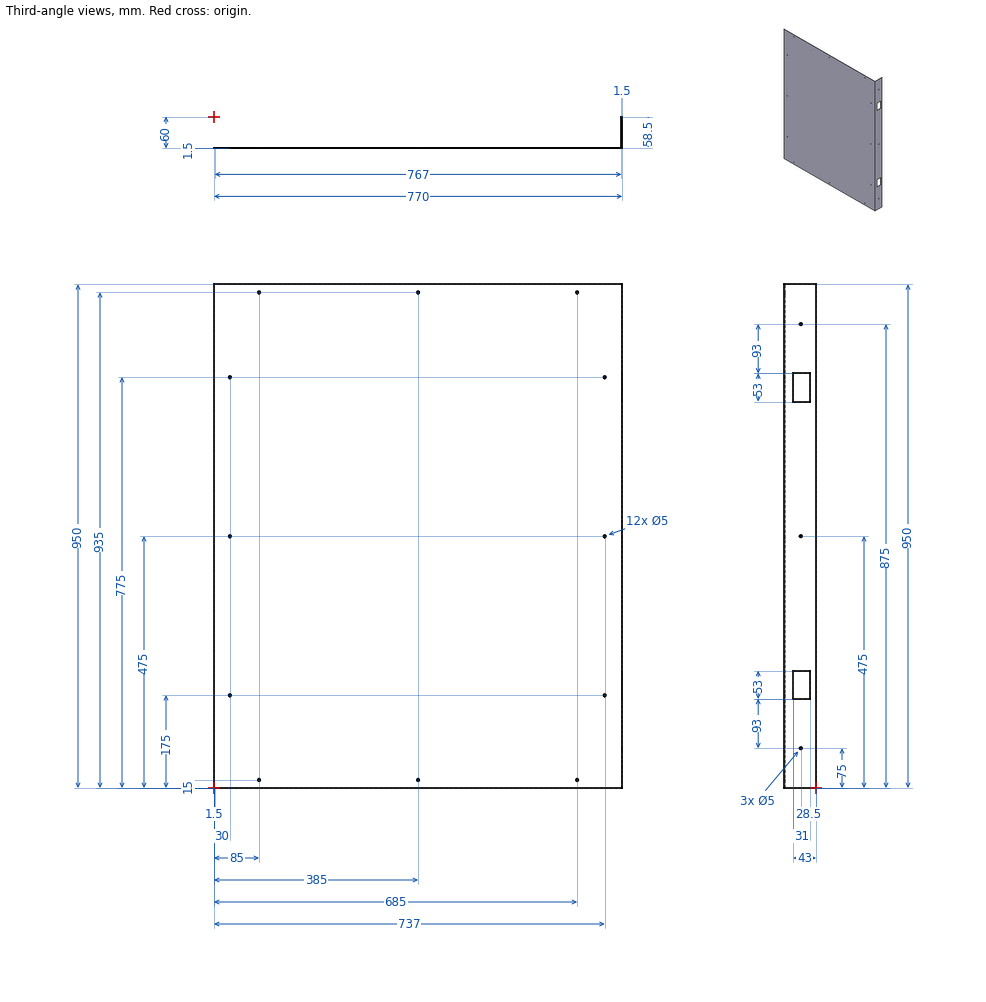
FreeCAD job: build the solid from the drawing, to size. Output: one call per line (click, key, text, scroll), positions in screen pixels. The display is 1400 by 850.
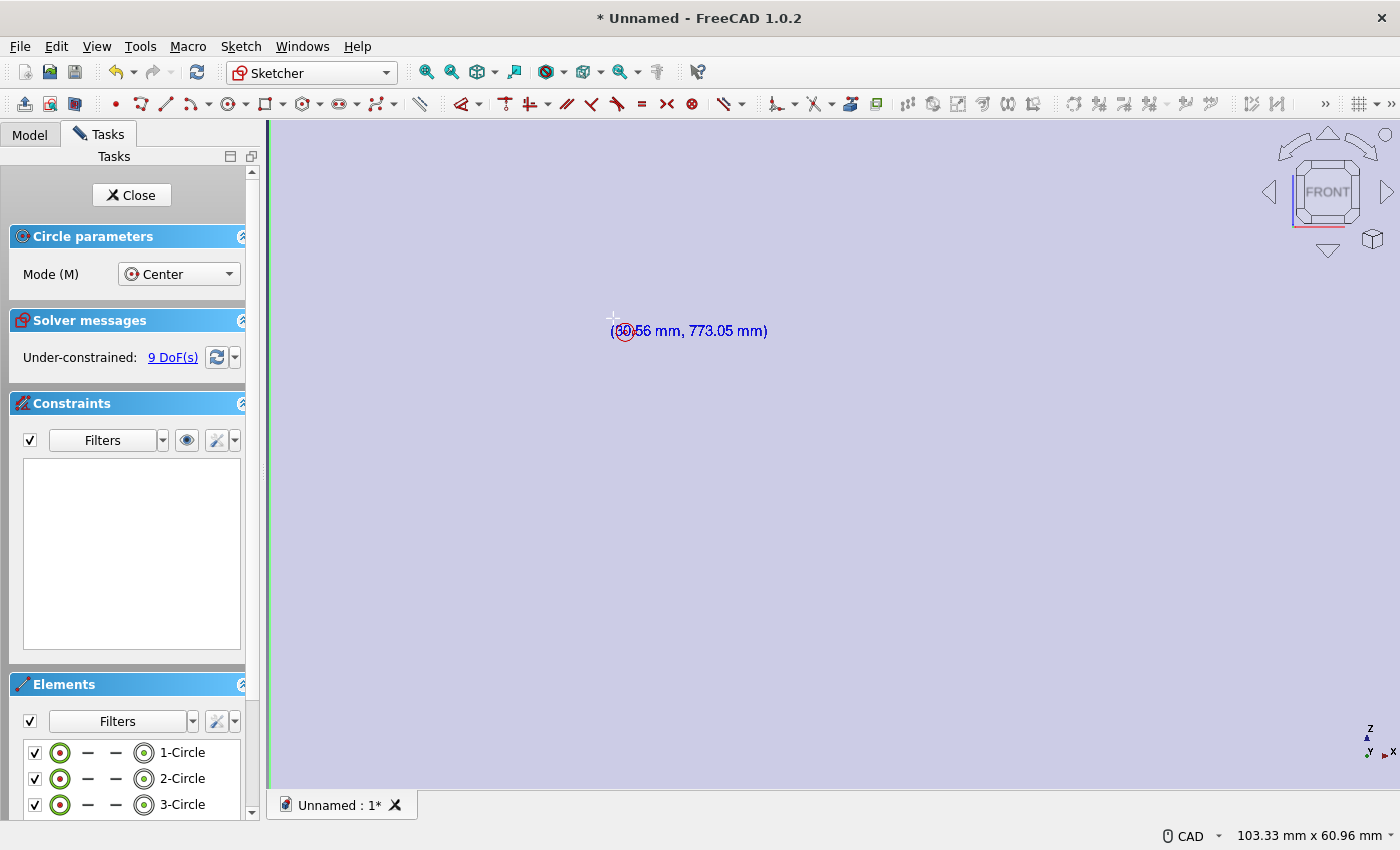
scroll(578, 286, down, 15)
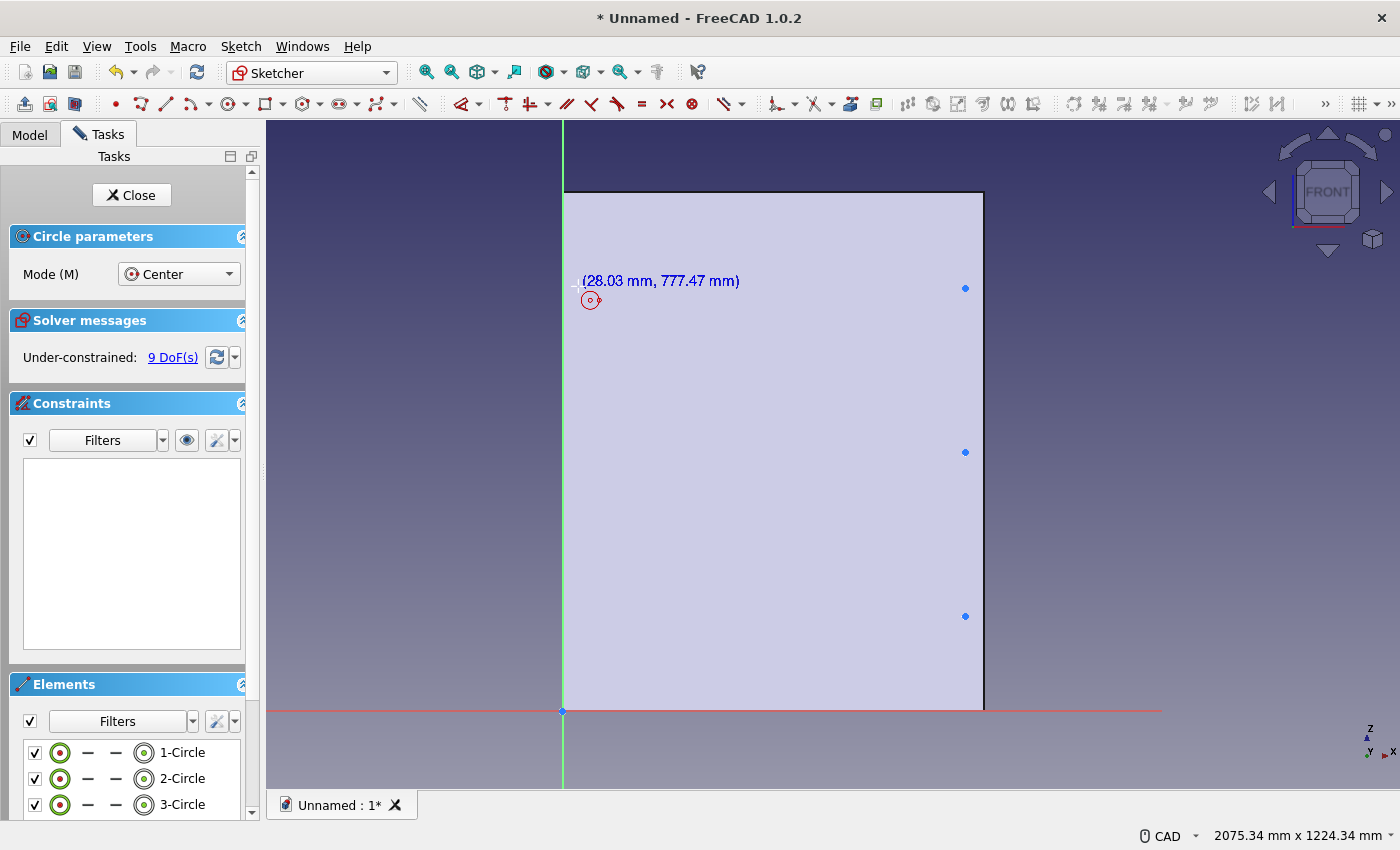
click(579, 288)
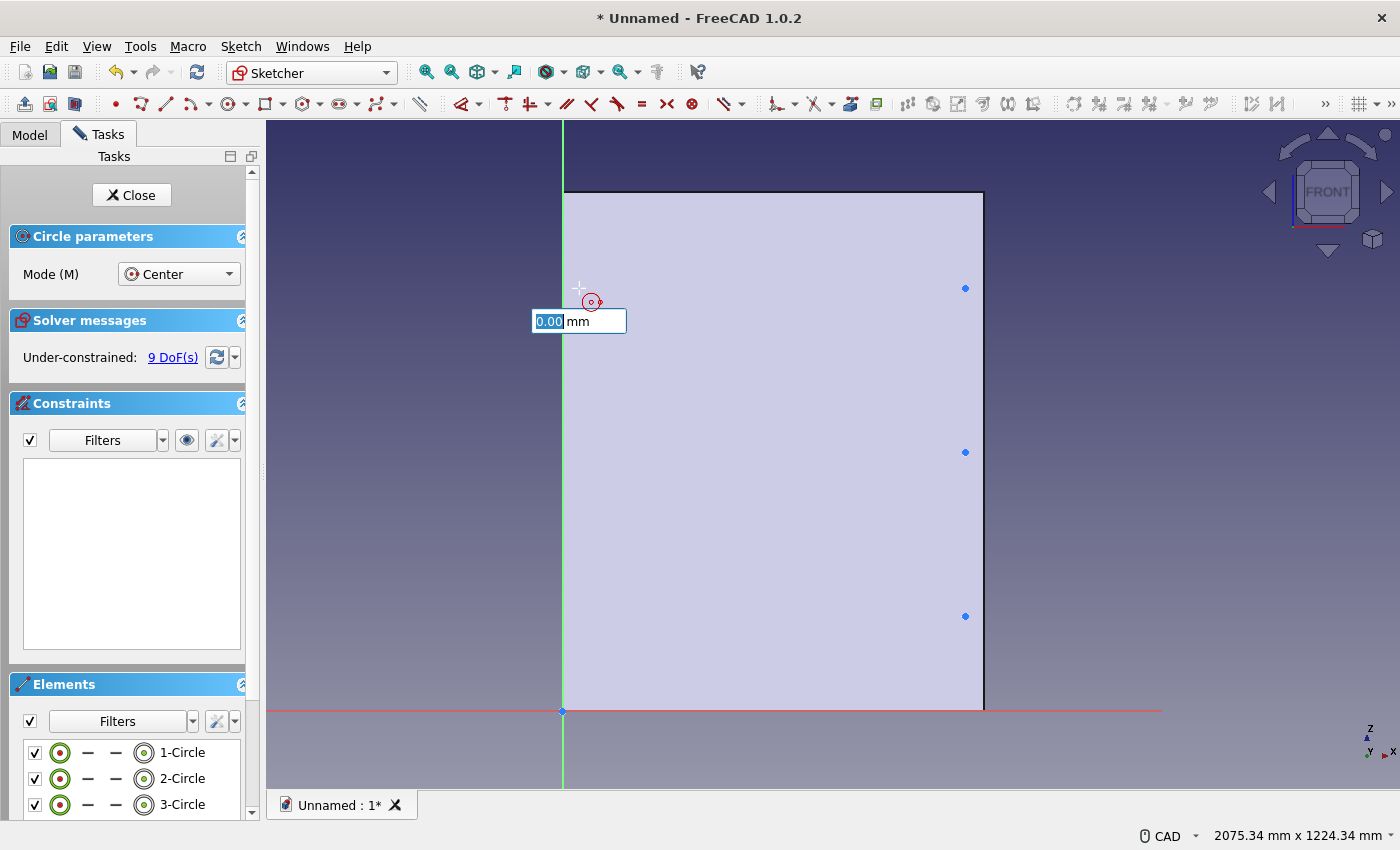
scroll(580, 287, up, 13)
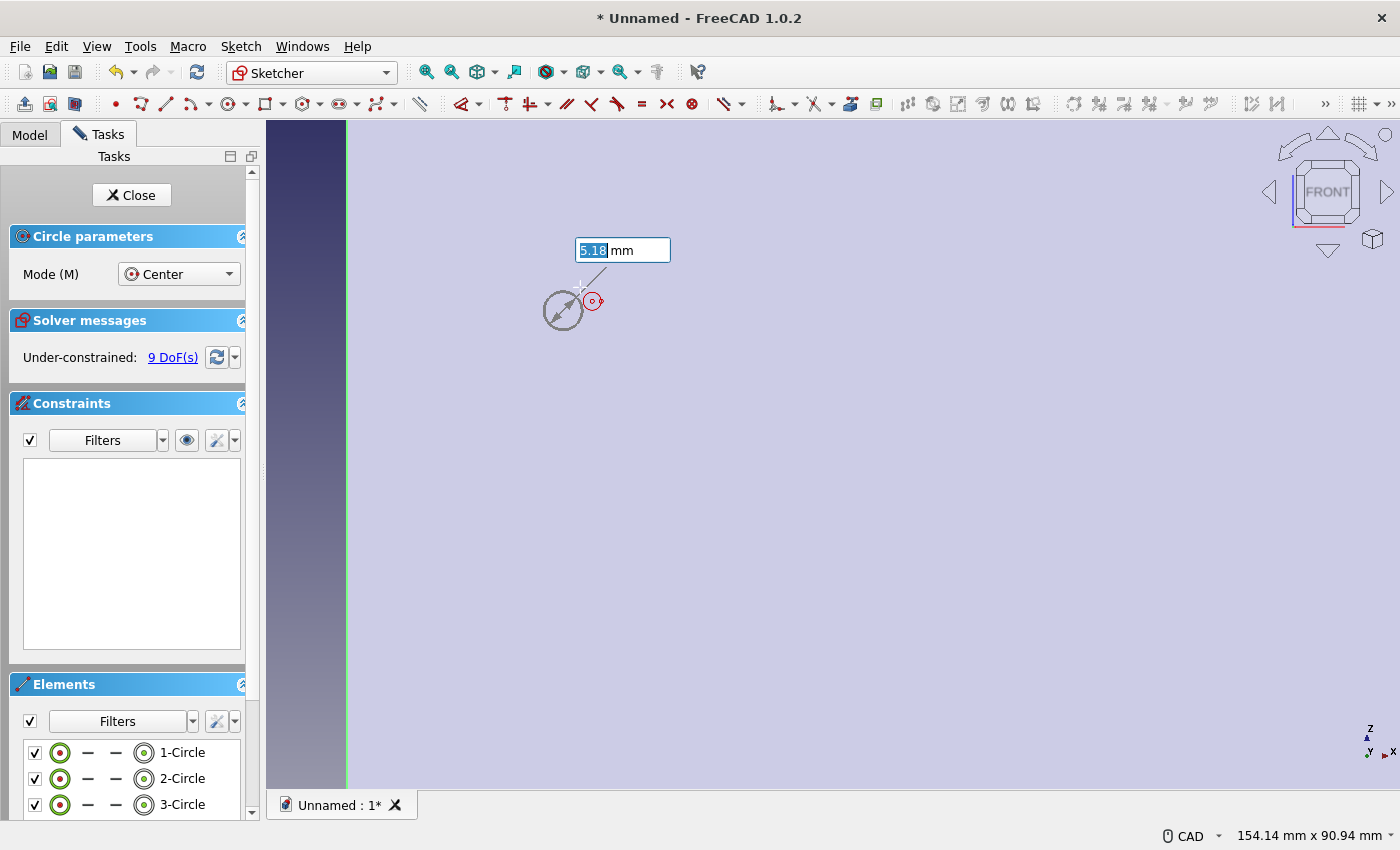
click(581, 279)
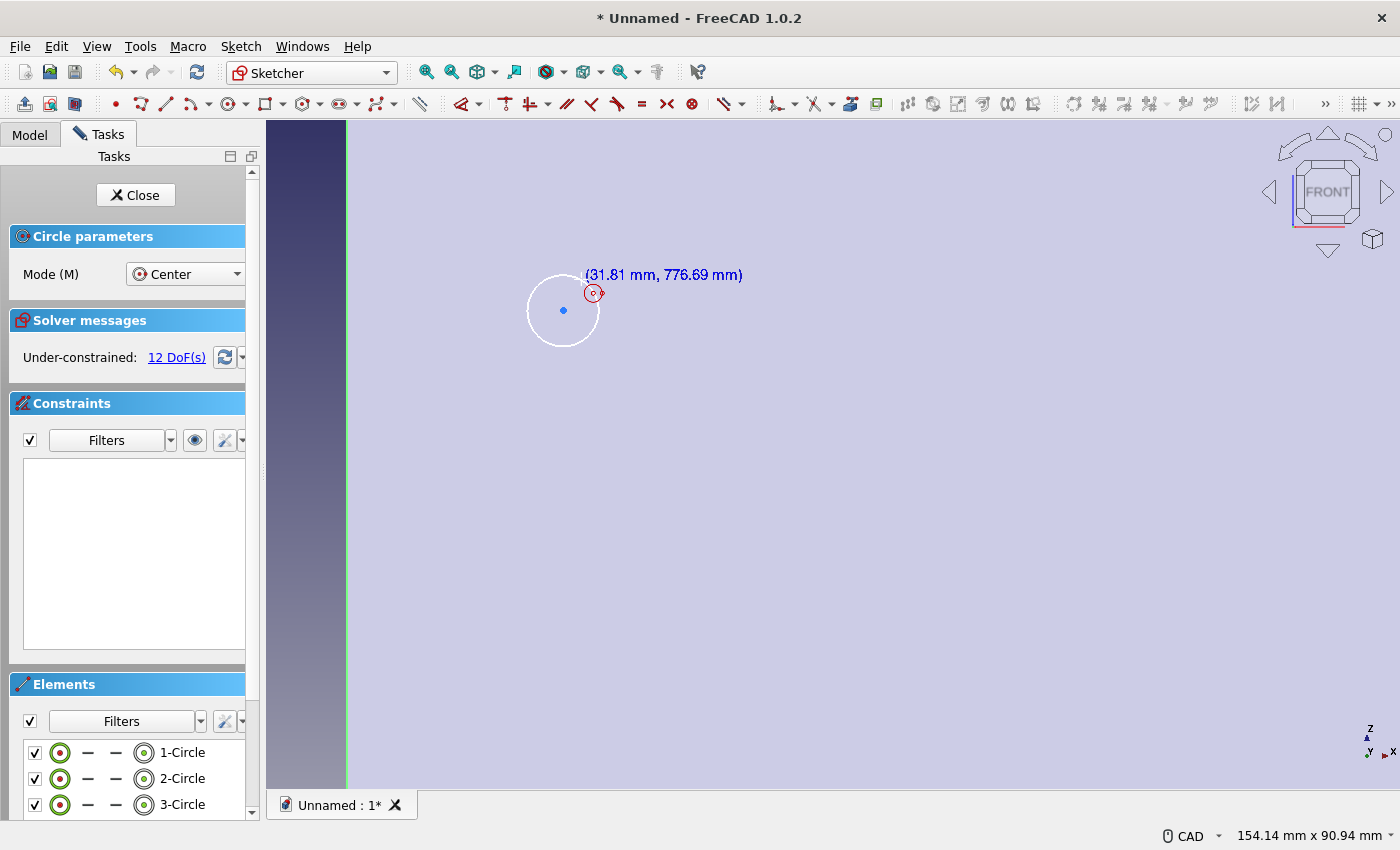
scroll(615, 319, down, 14)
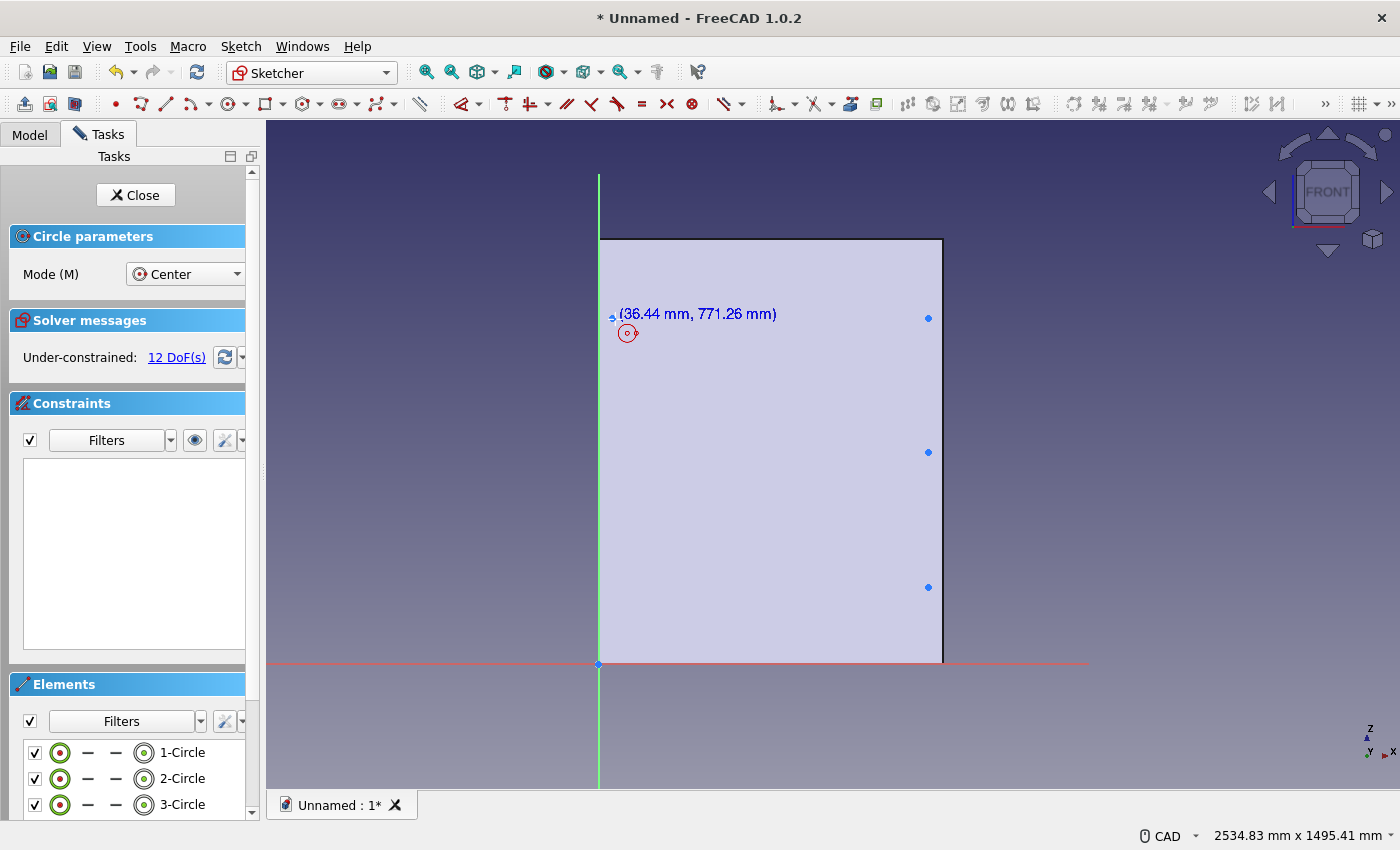
scroll(612, 452, up, 16)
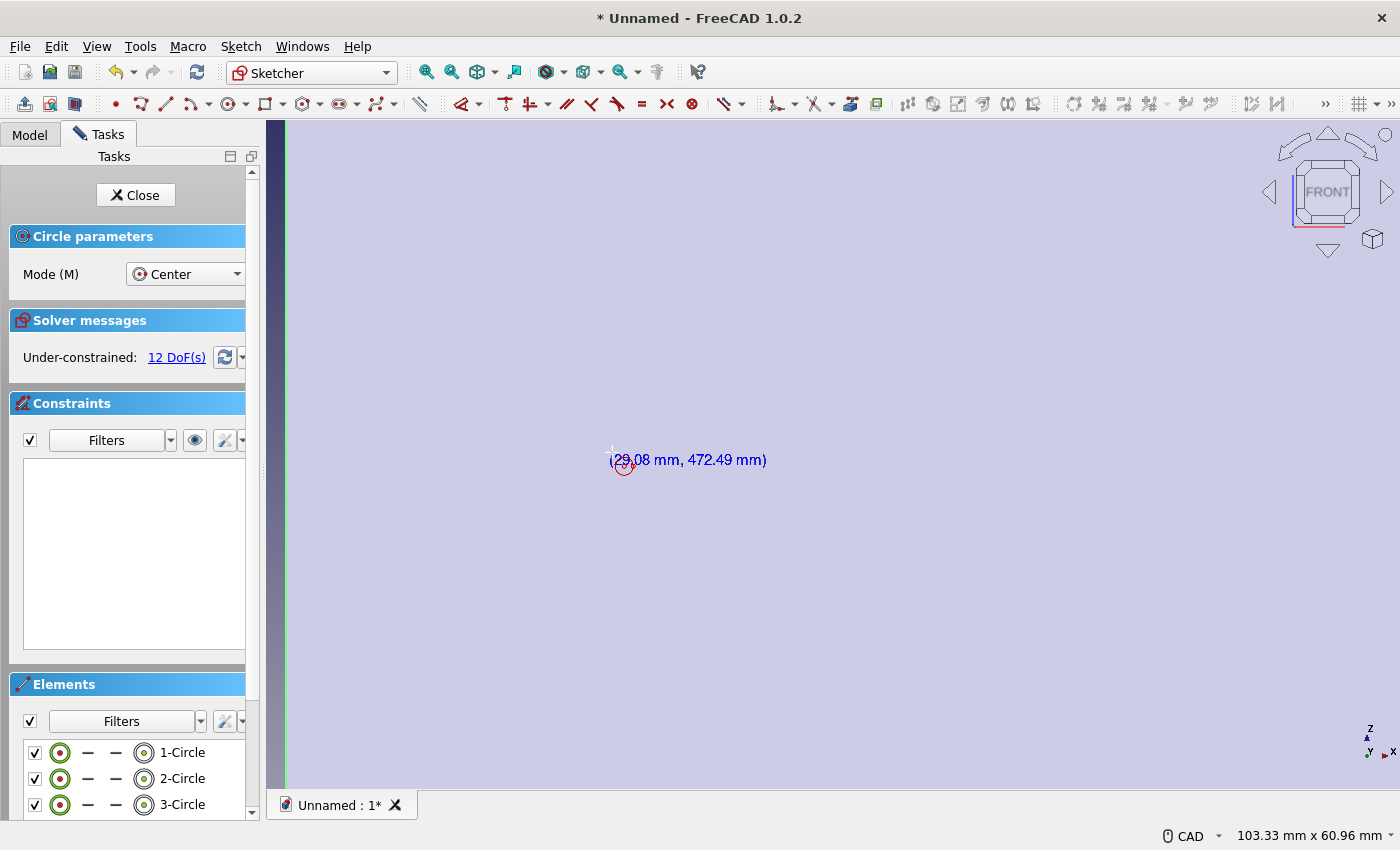
scroll(577, 452, down, 15)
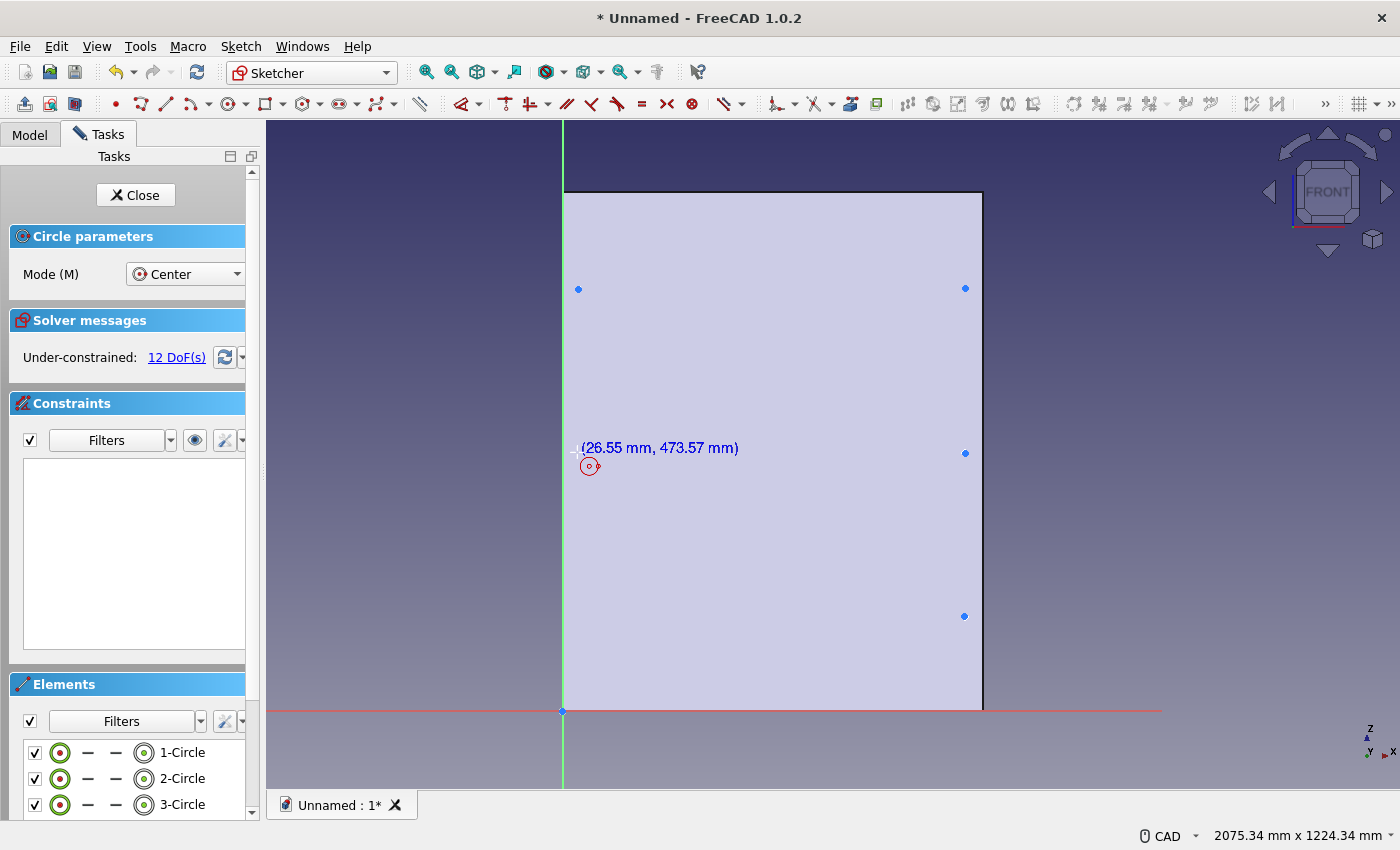
click(579, 452)